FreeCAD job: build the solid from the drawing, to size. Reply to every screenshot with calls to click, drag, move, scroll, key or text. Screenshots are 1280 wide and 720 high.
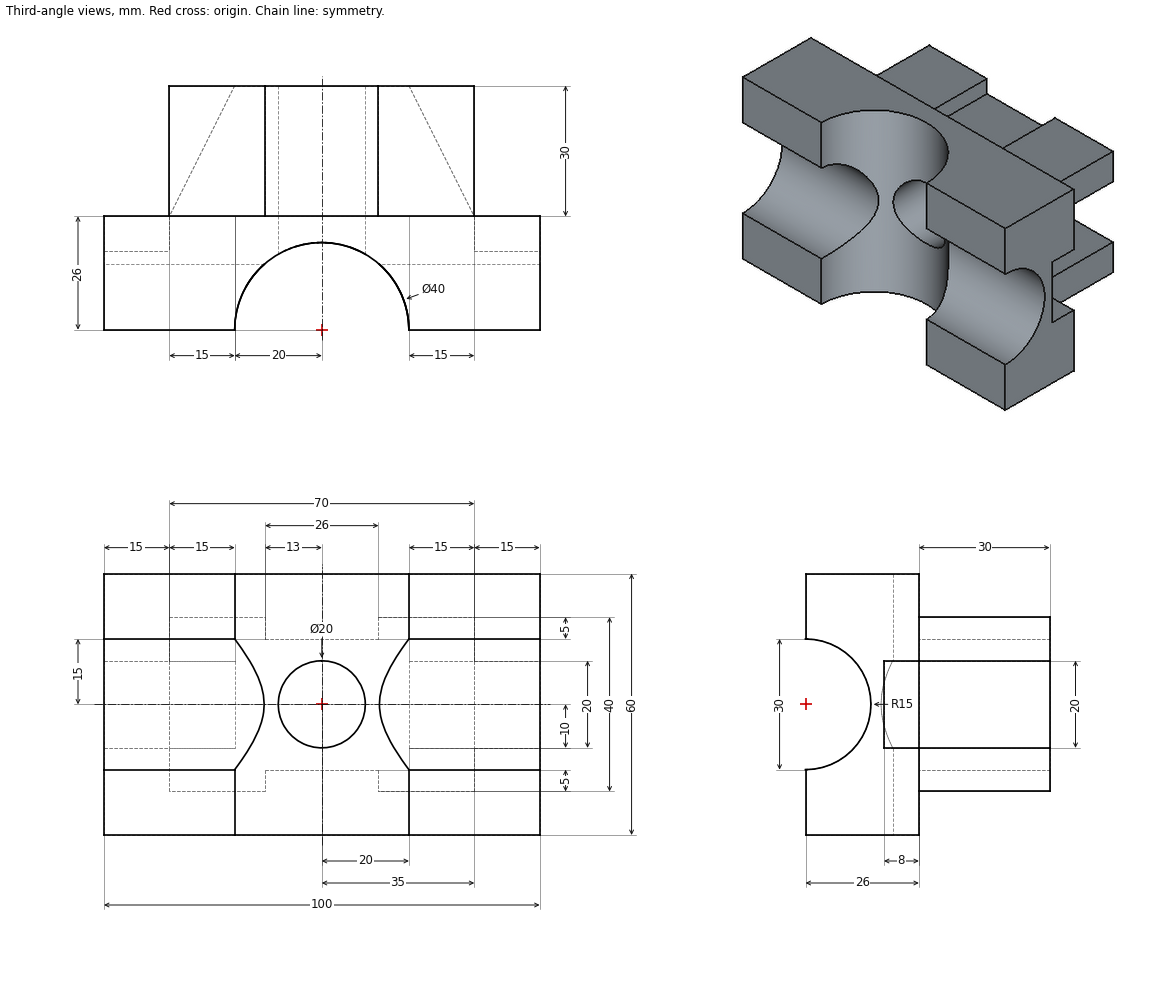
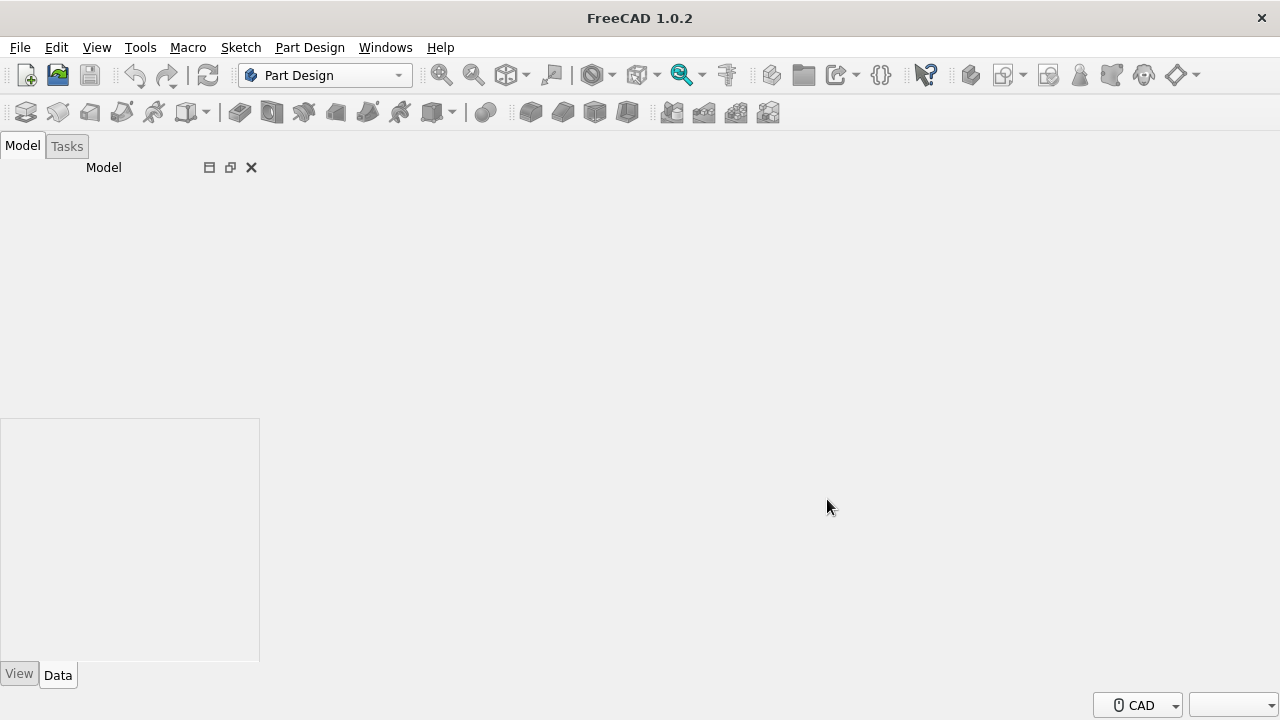
click(26, 76)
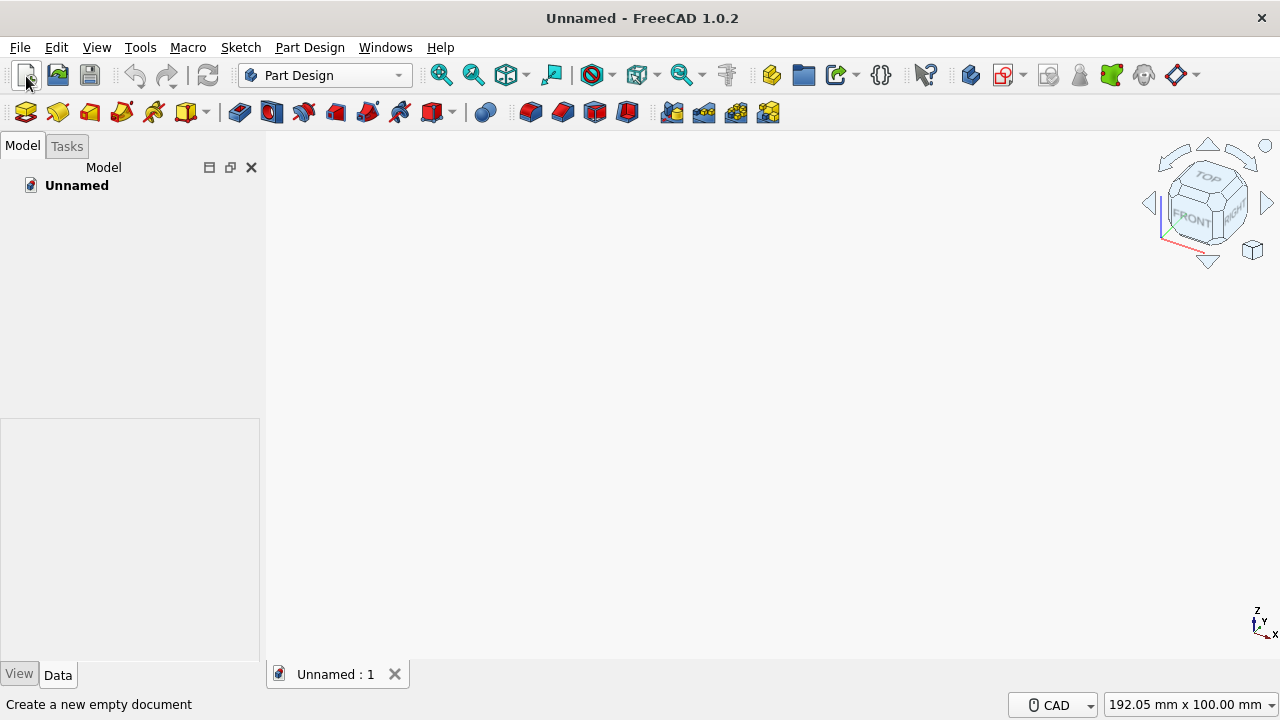
click(1004, 76)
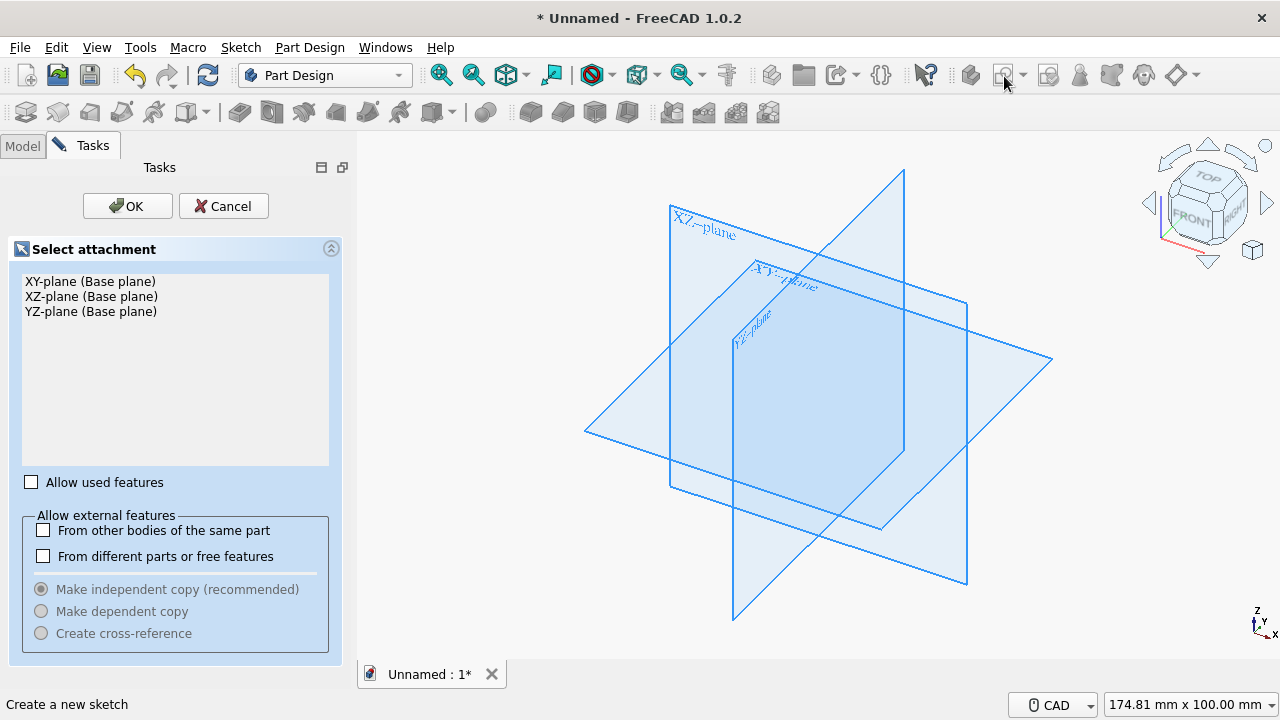
click(82, 296)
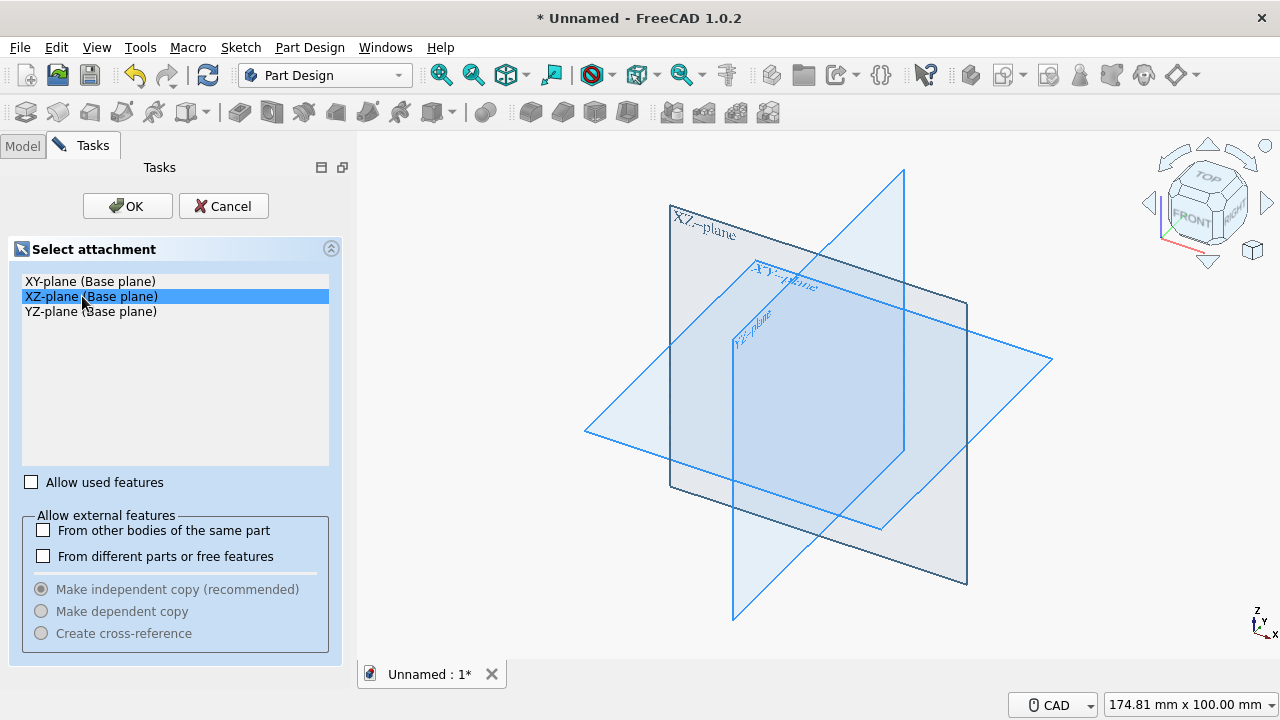
click(128, 206)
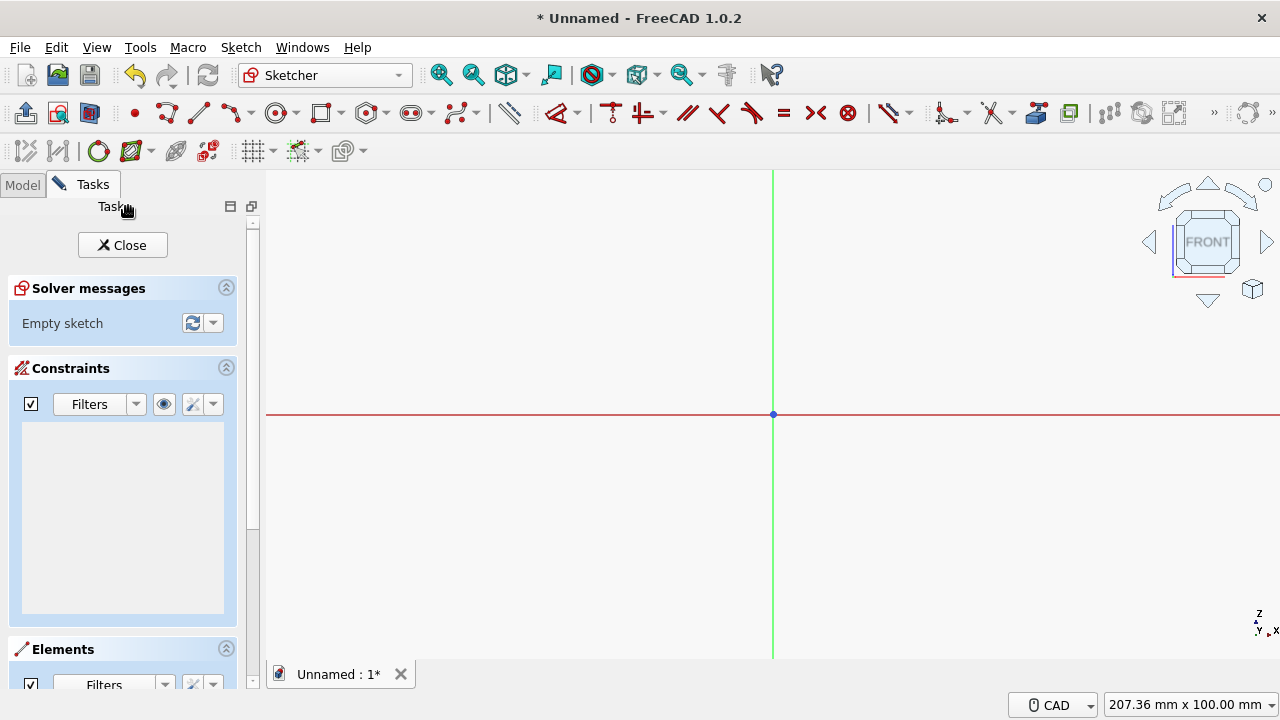
key(g)
key(v)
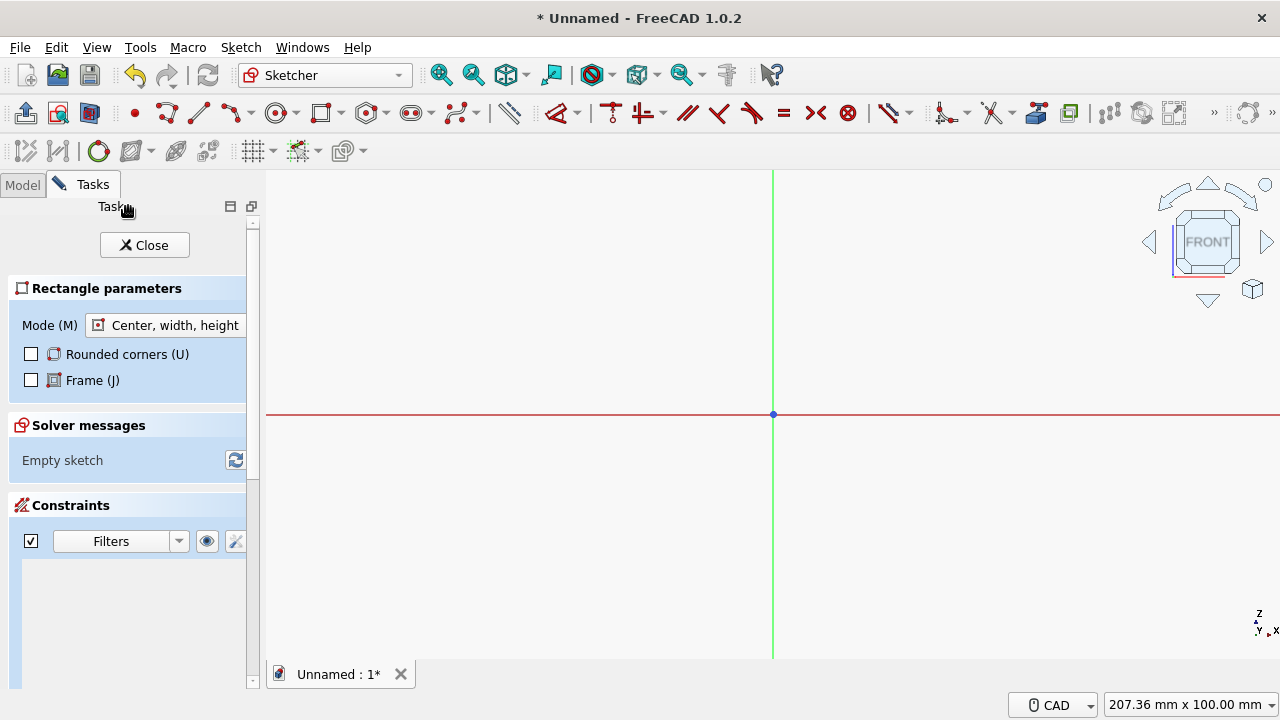
click(773, 414)
move(1018, 268)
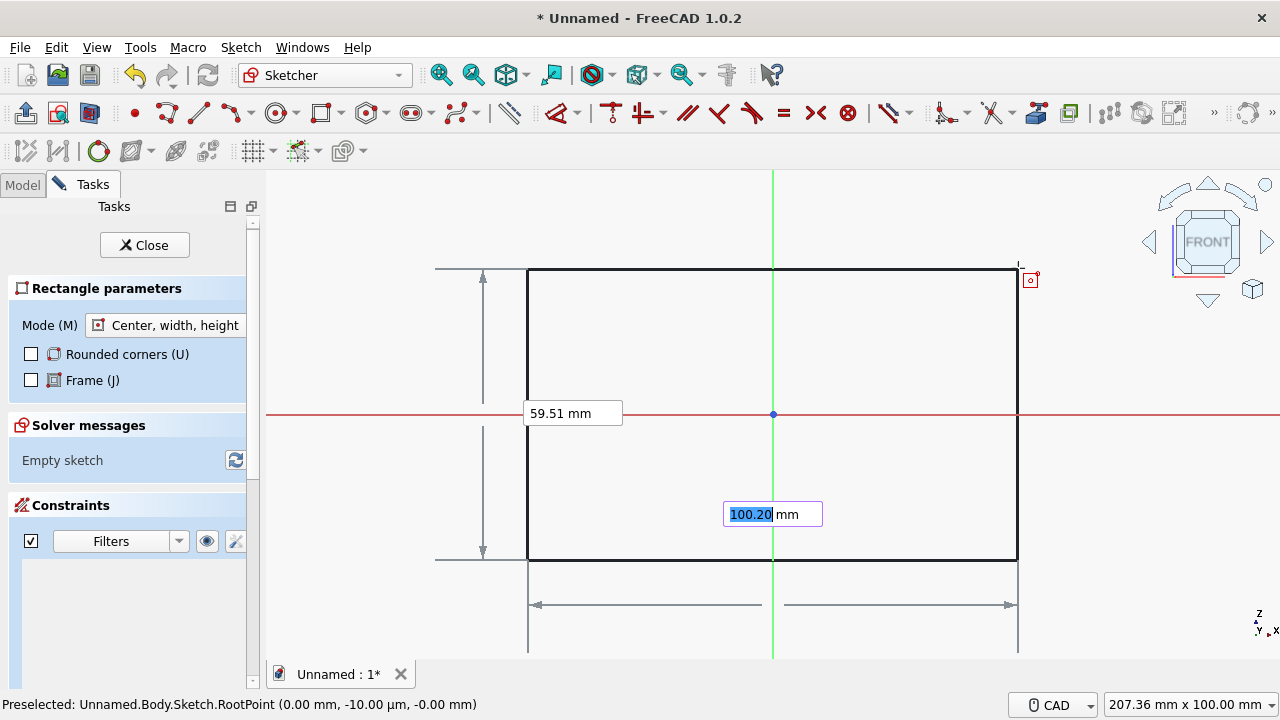
text(100)
key(Tab)
text(60)
key(Return)
key(Escape)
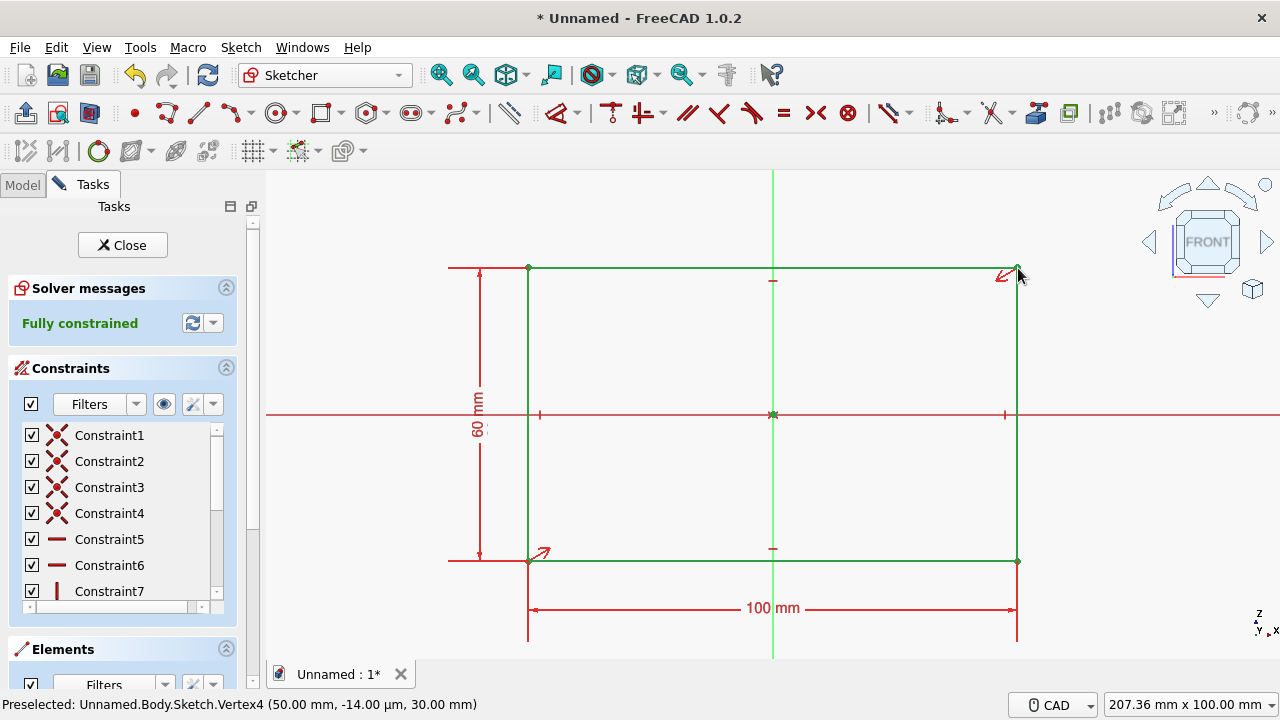
click(123, 245)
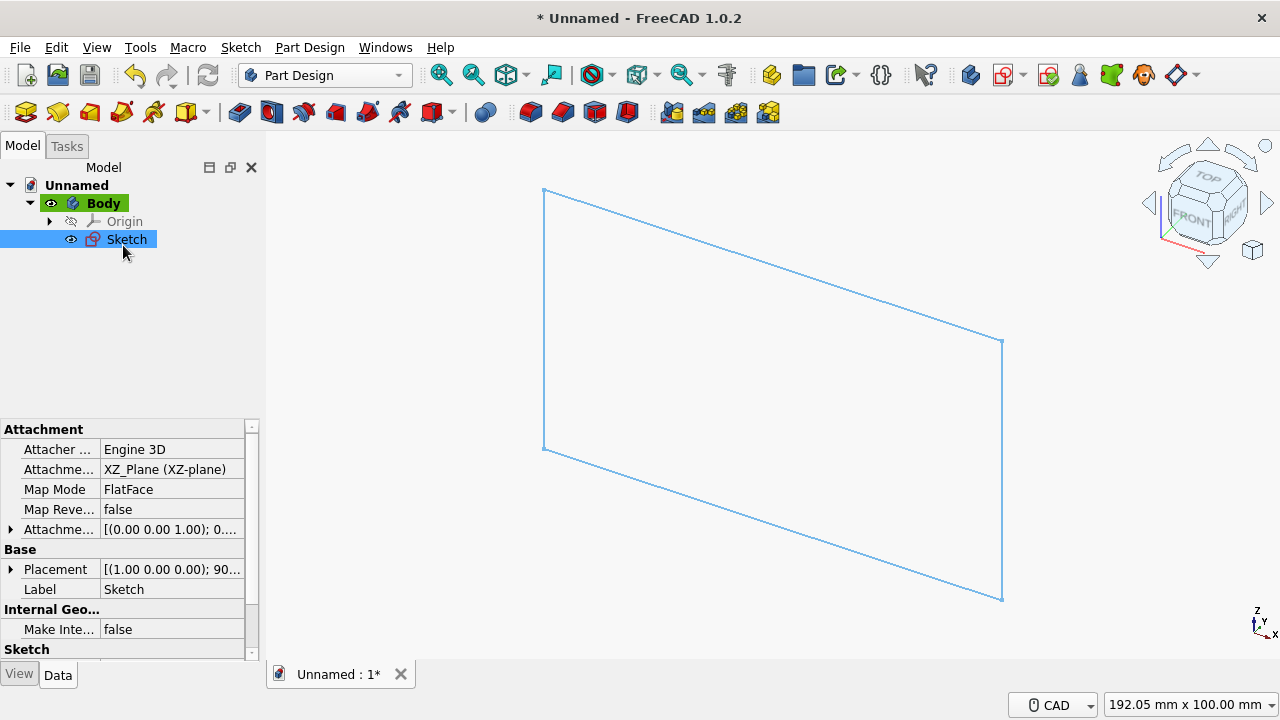
click(26, 112)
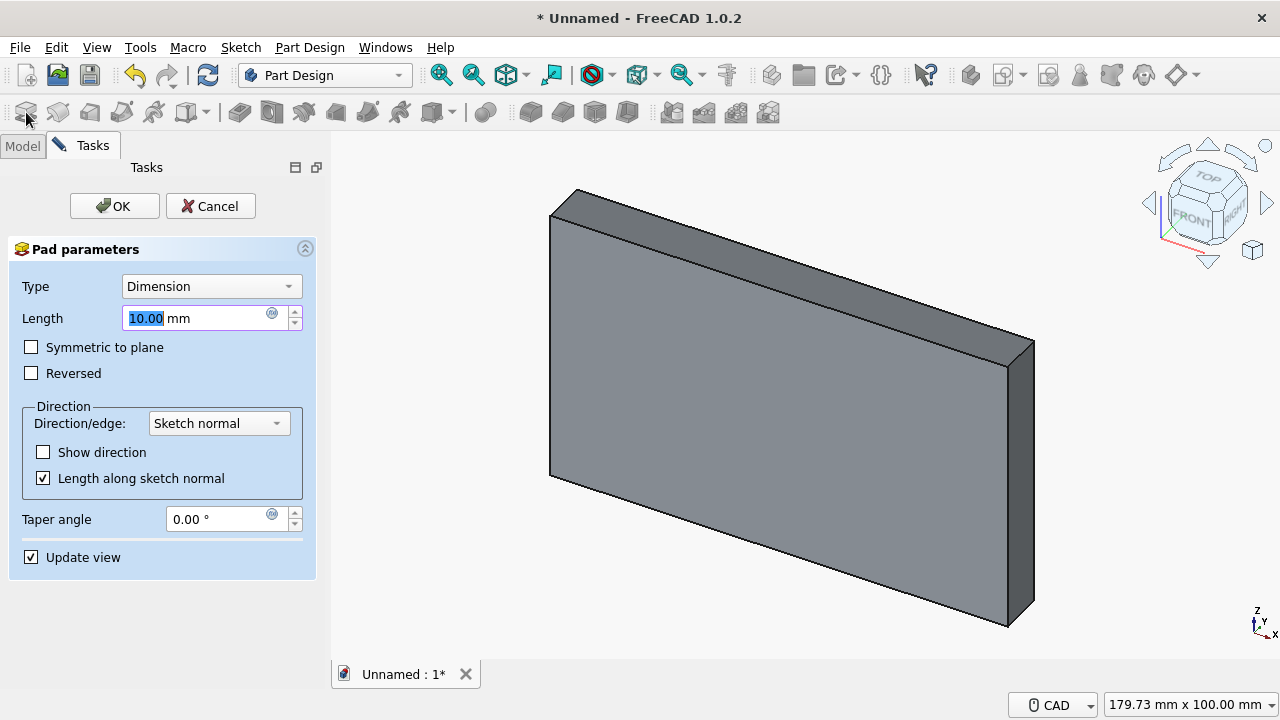
text(26)
key(Tab)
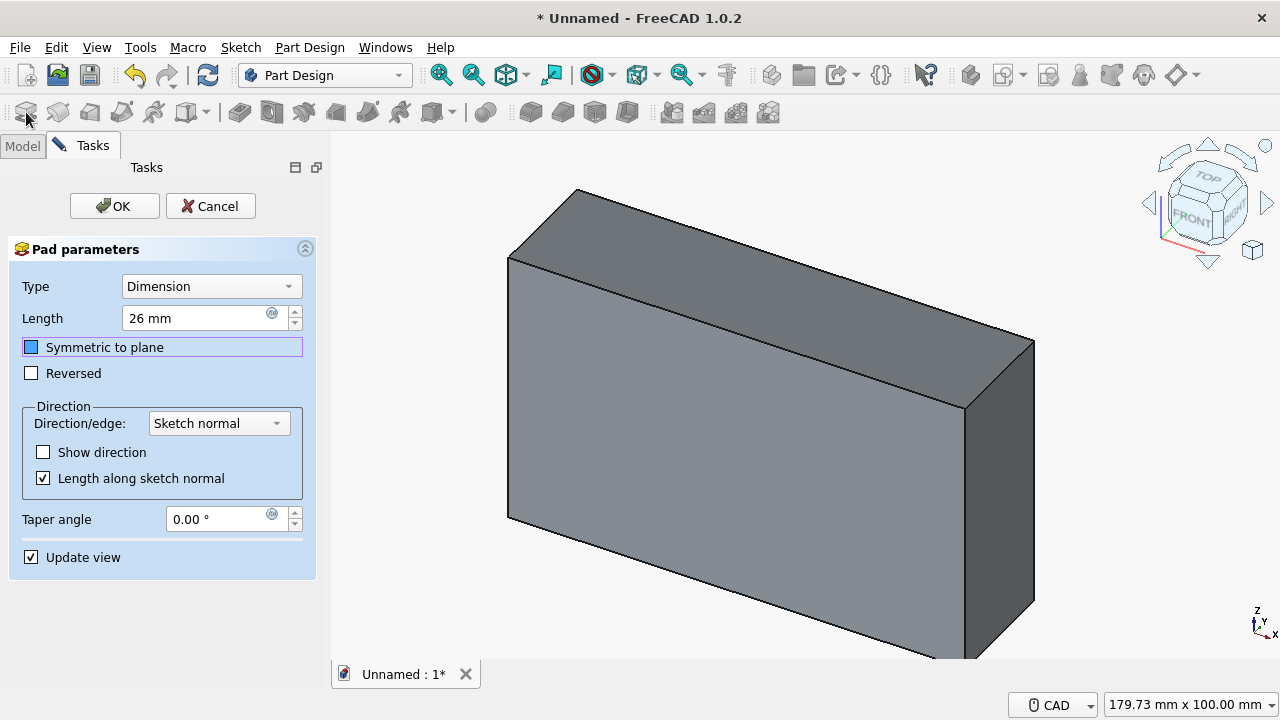
click(30, 373)